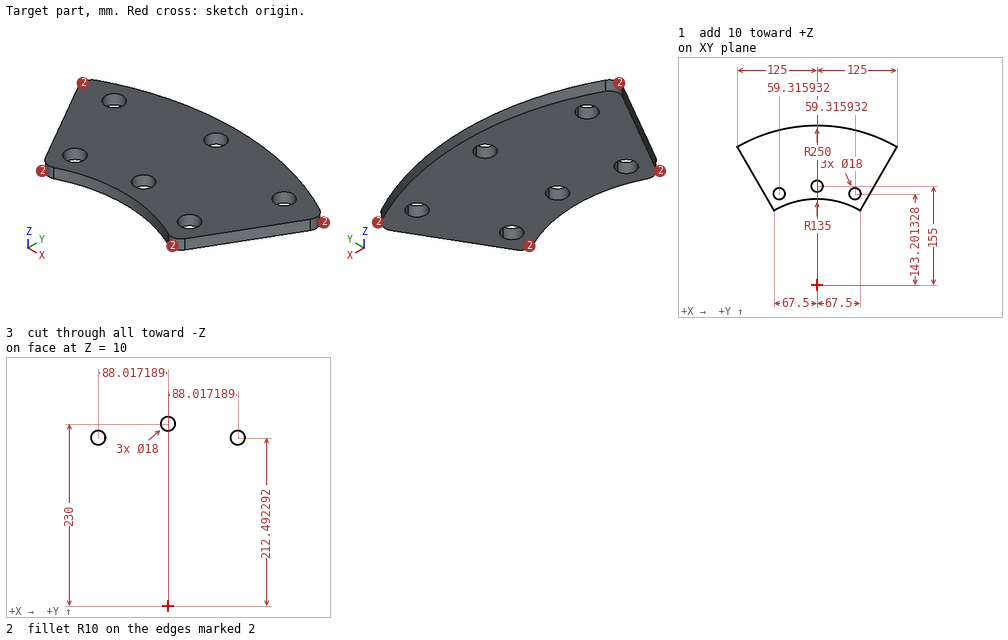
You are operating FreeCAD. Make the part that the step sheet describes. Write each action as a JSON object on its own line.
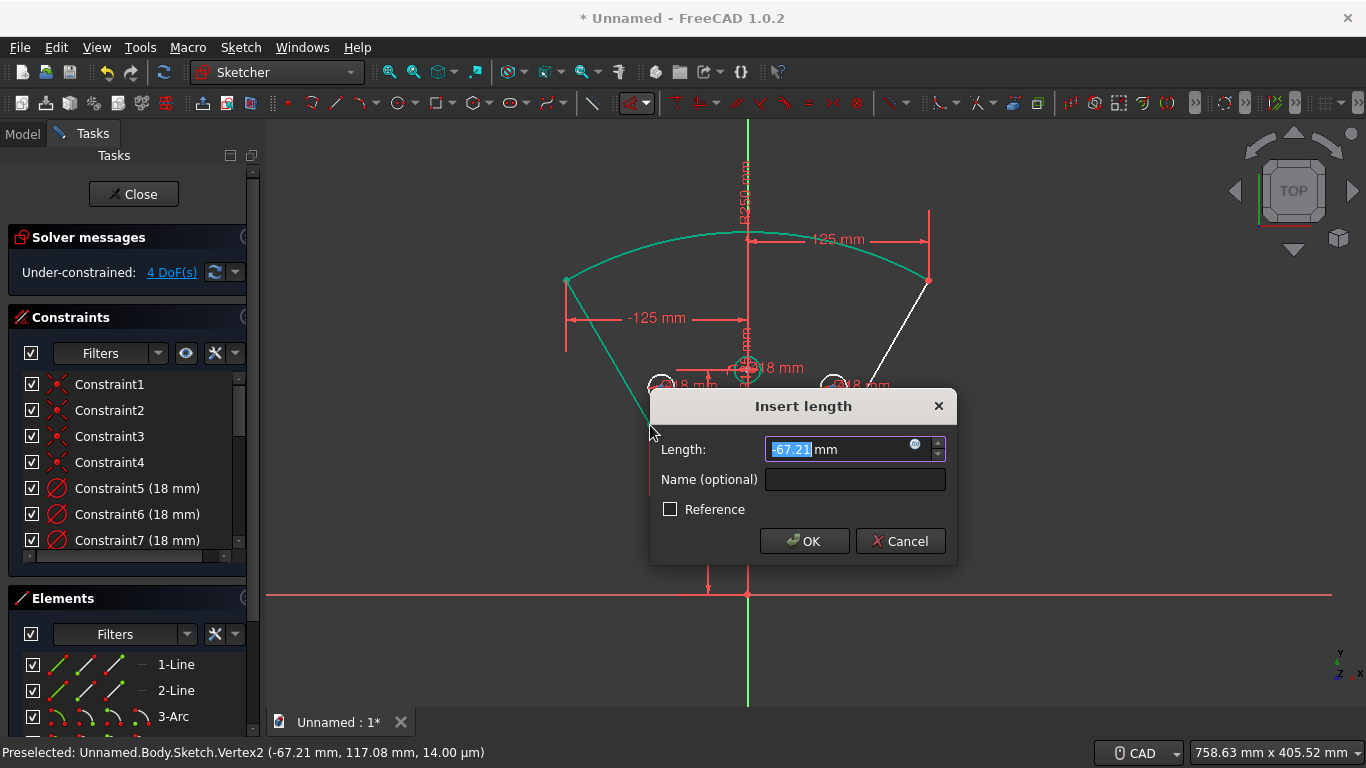
{"action": "type", "text": "-67.5"}
{"action": "key", "text": "Return"}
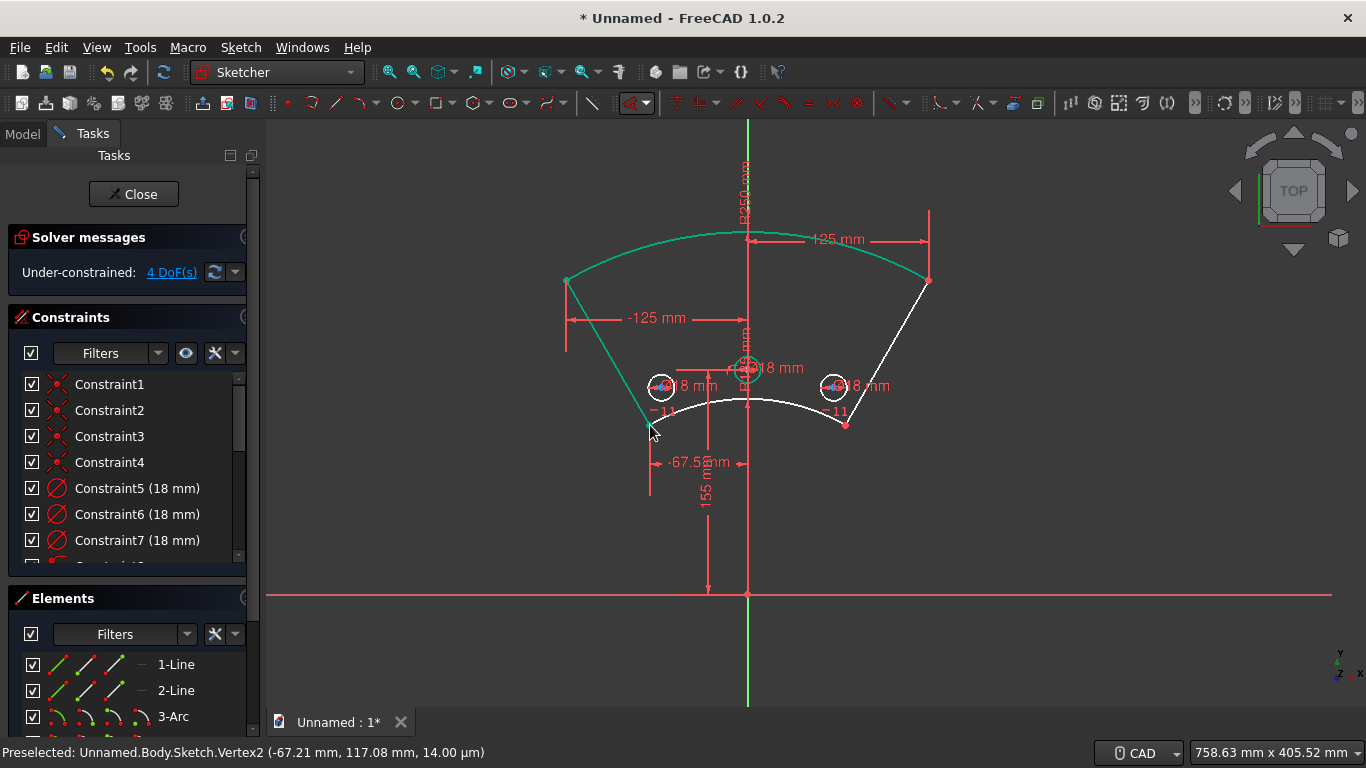
{"action": "left_click", "coordinate": [845, 425]}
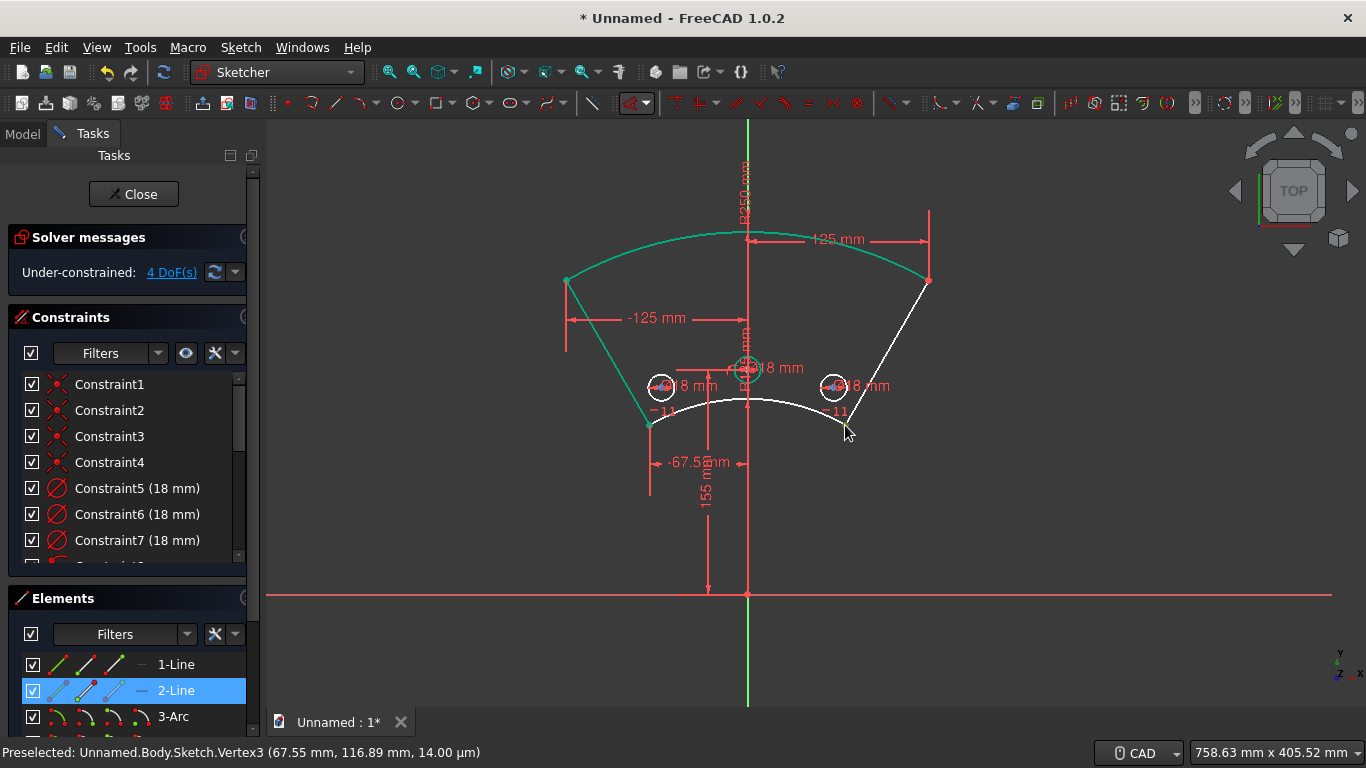
{"action": "left_click", "coordinate": [648, 104]}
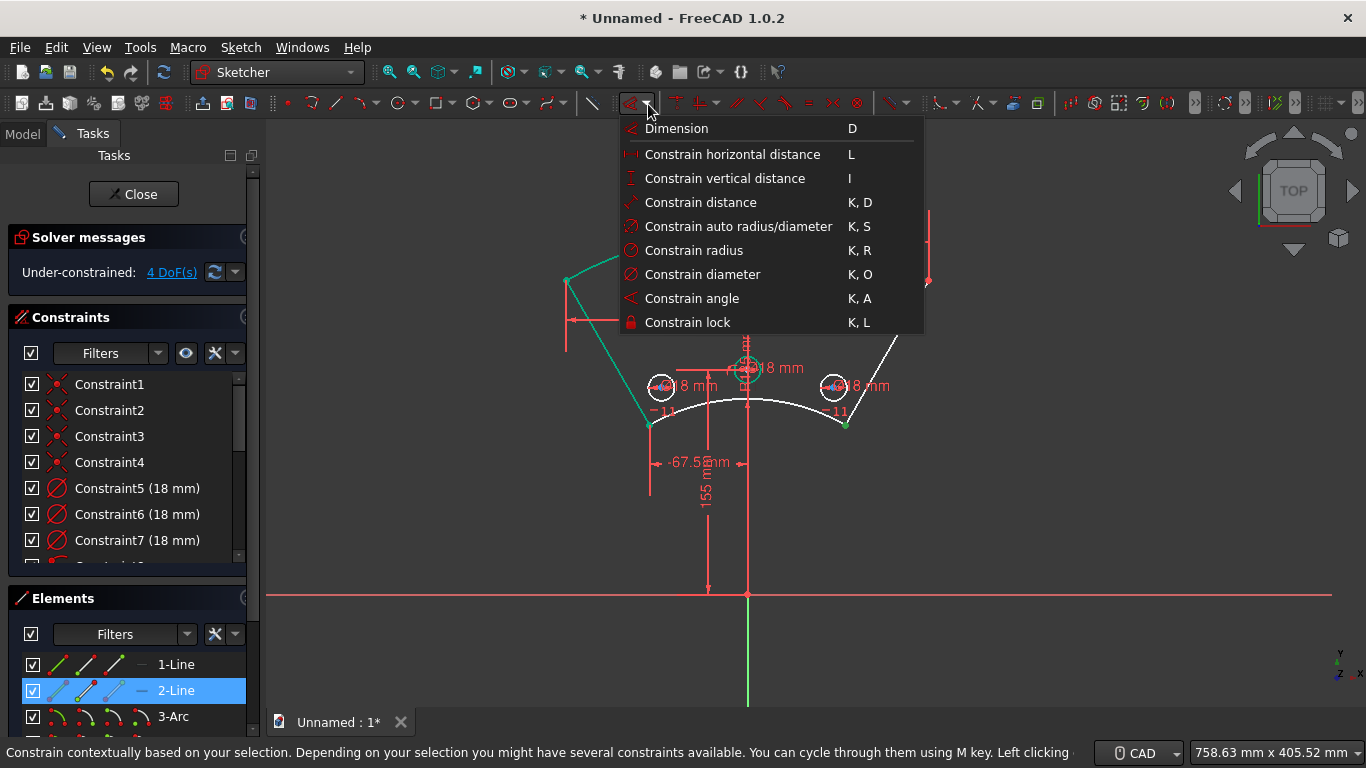
{"action": "left_click", "coordinate": [772, 154]}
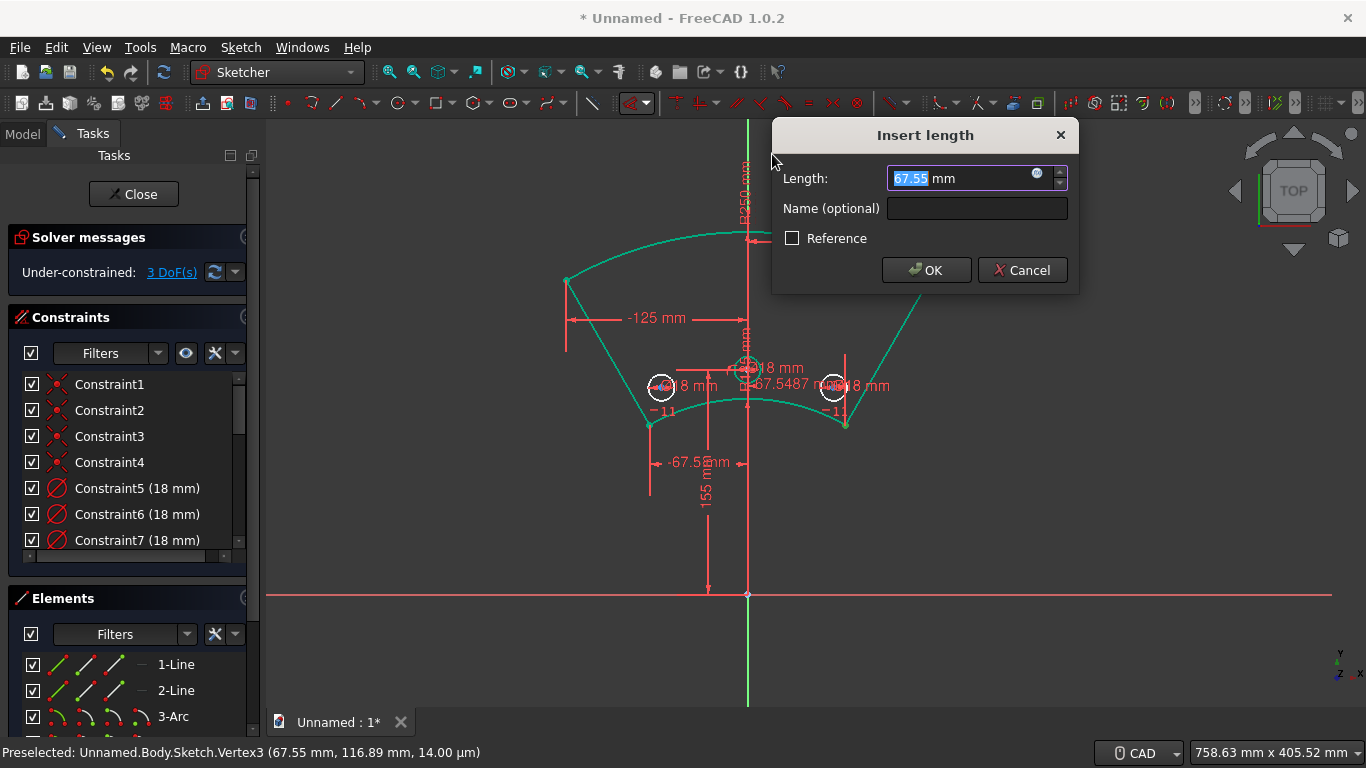
{"action": "type", "text": "67.5"}
{"action": "key", "text": "Return"}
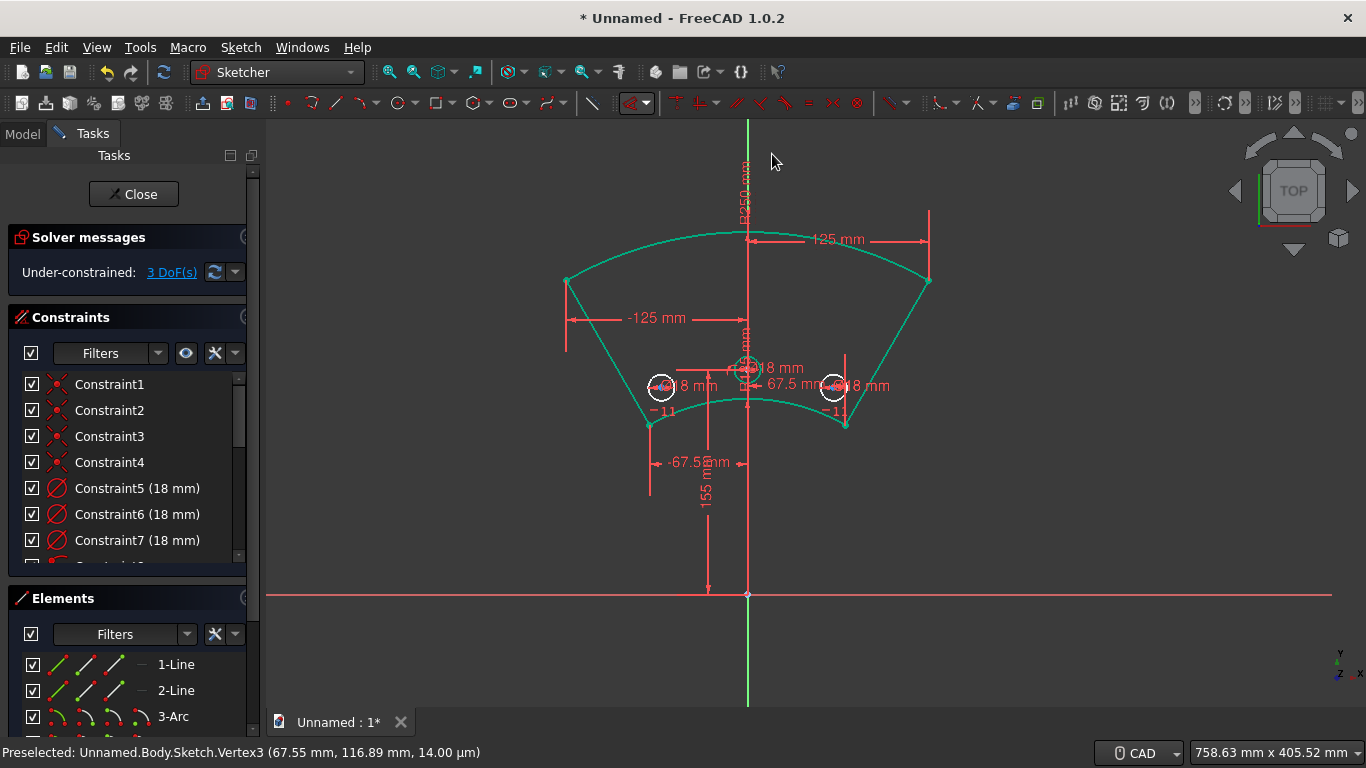
{"action": "left_click", "coordinate": [834, 388]}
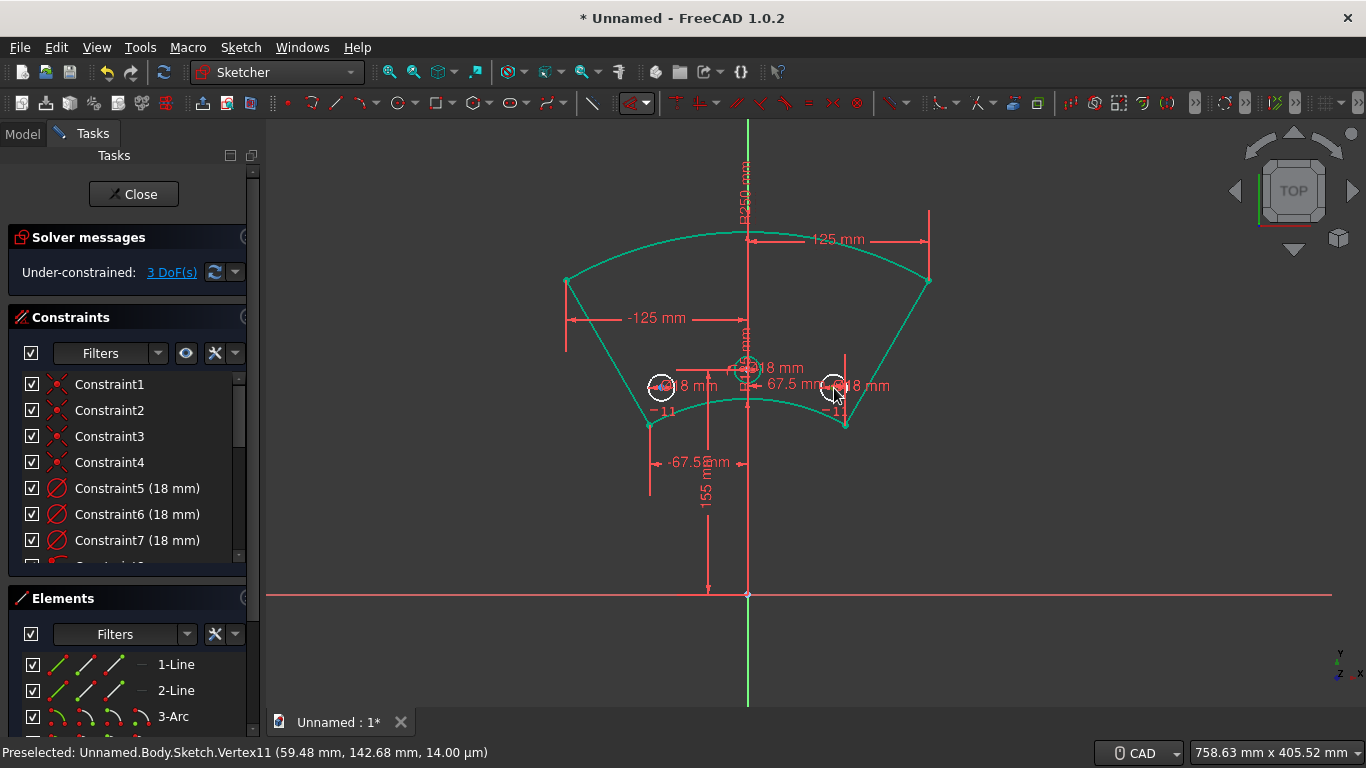
{"action": "key", "text": "l"}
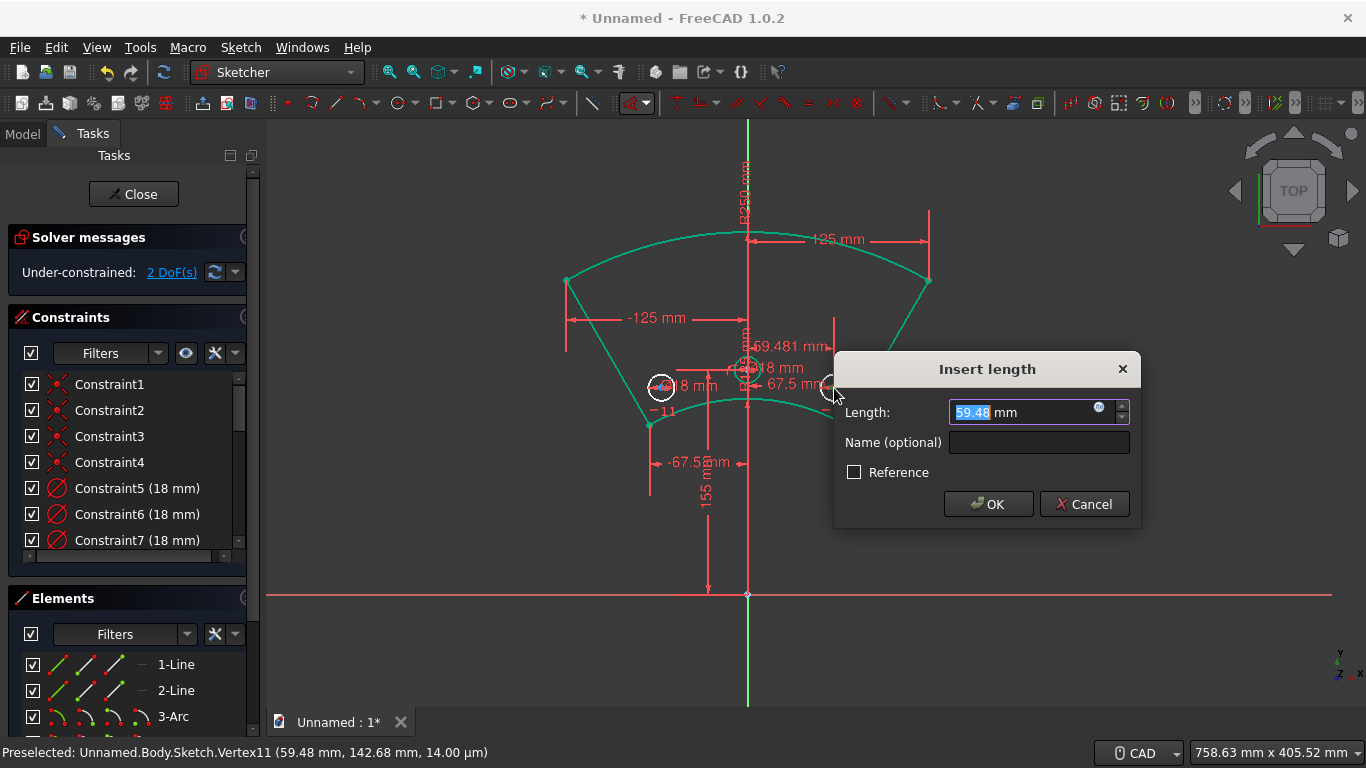
{"action": "type", "text": "59.315932"}
{"action": "key", "text": "Return"}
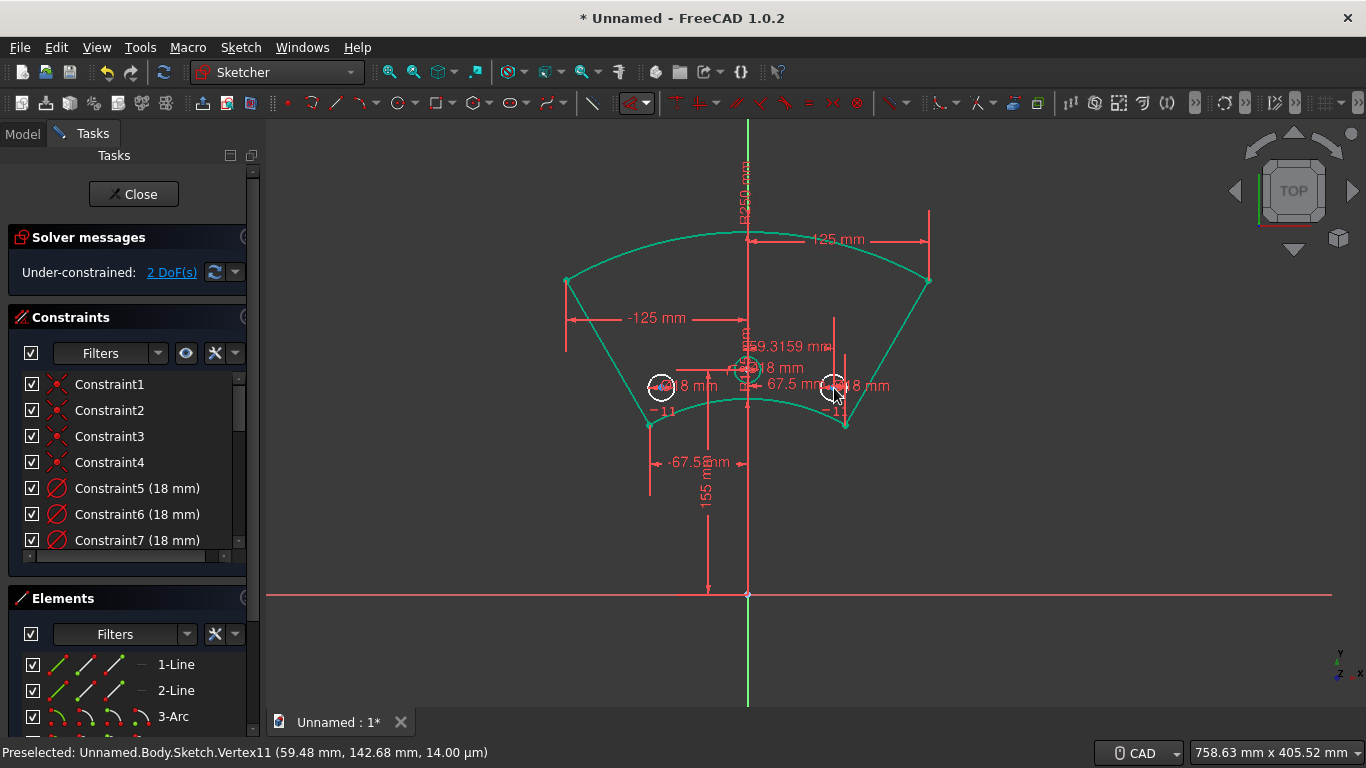
{"action": "left_click", "coordinate": [661, 388]}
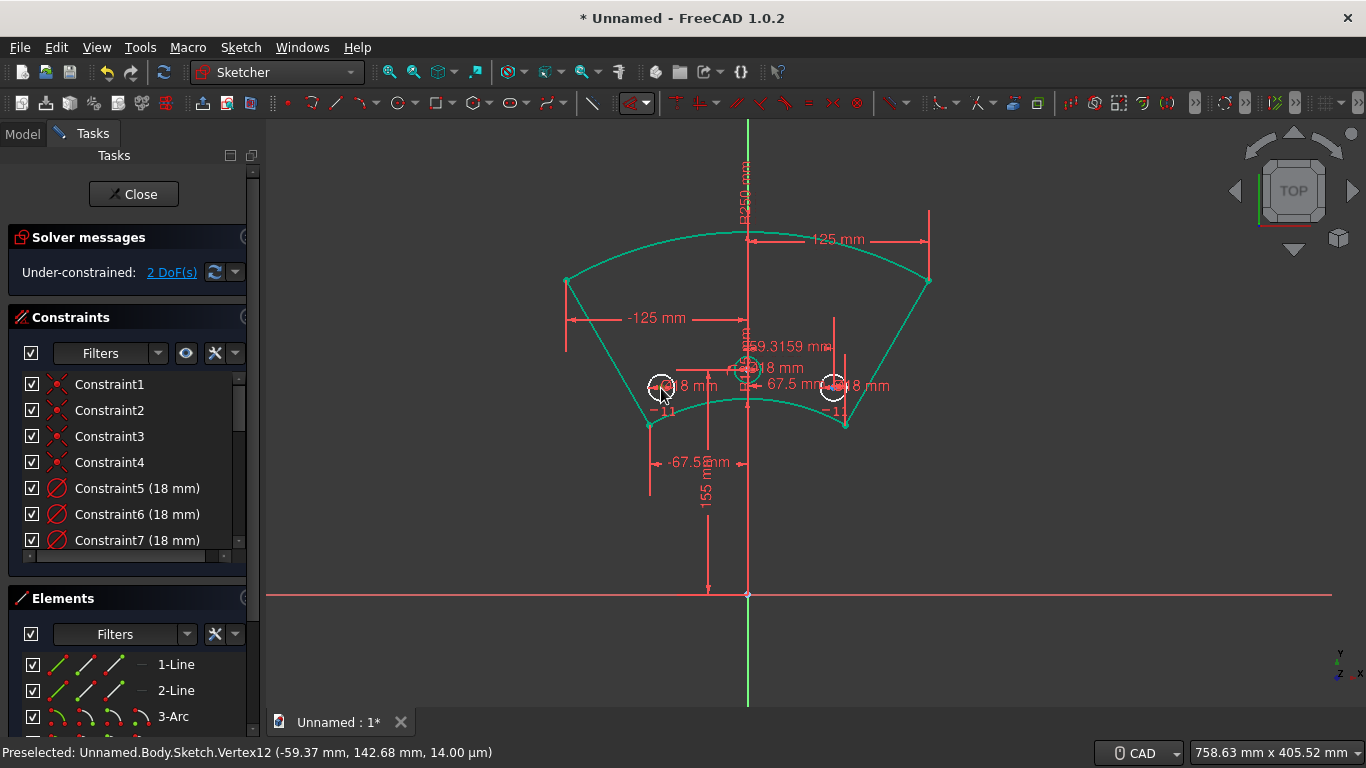
{"action": "key", "text": "l"}